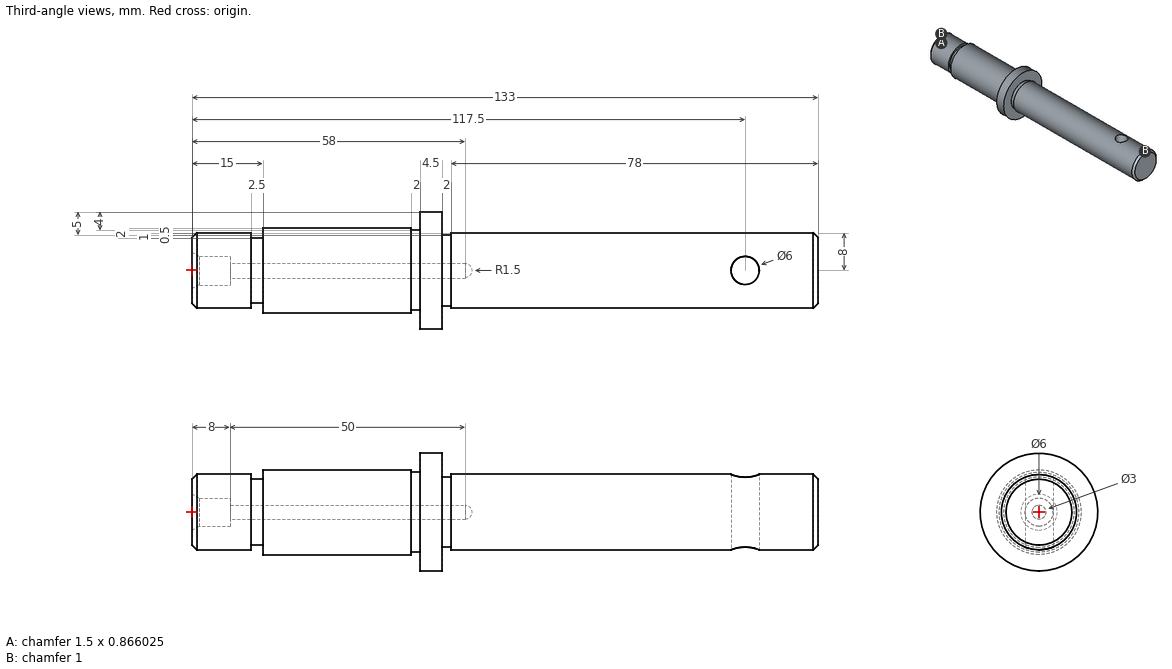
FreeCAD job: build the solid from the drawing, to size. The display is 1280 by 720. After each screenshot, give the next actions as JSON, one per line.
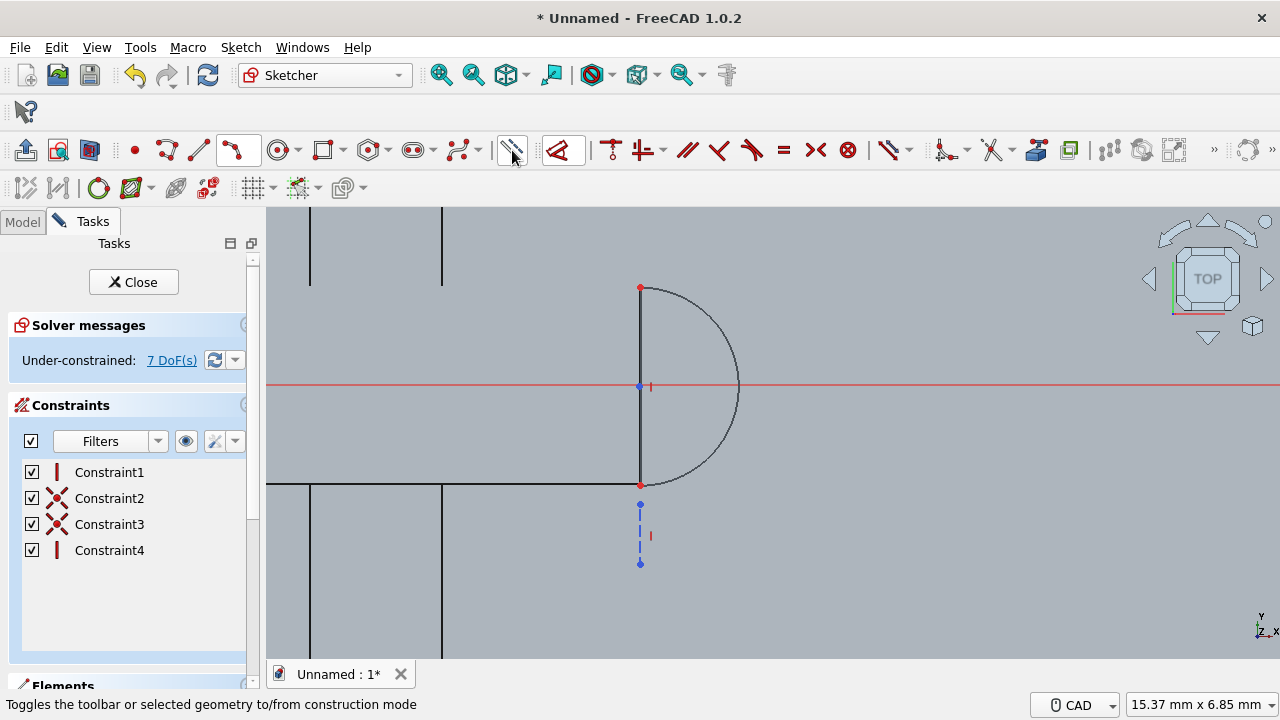
{"action": "left_click", "coordinate": [640, 387]}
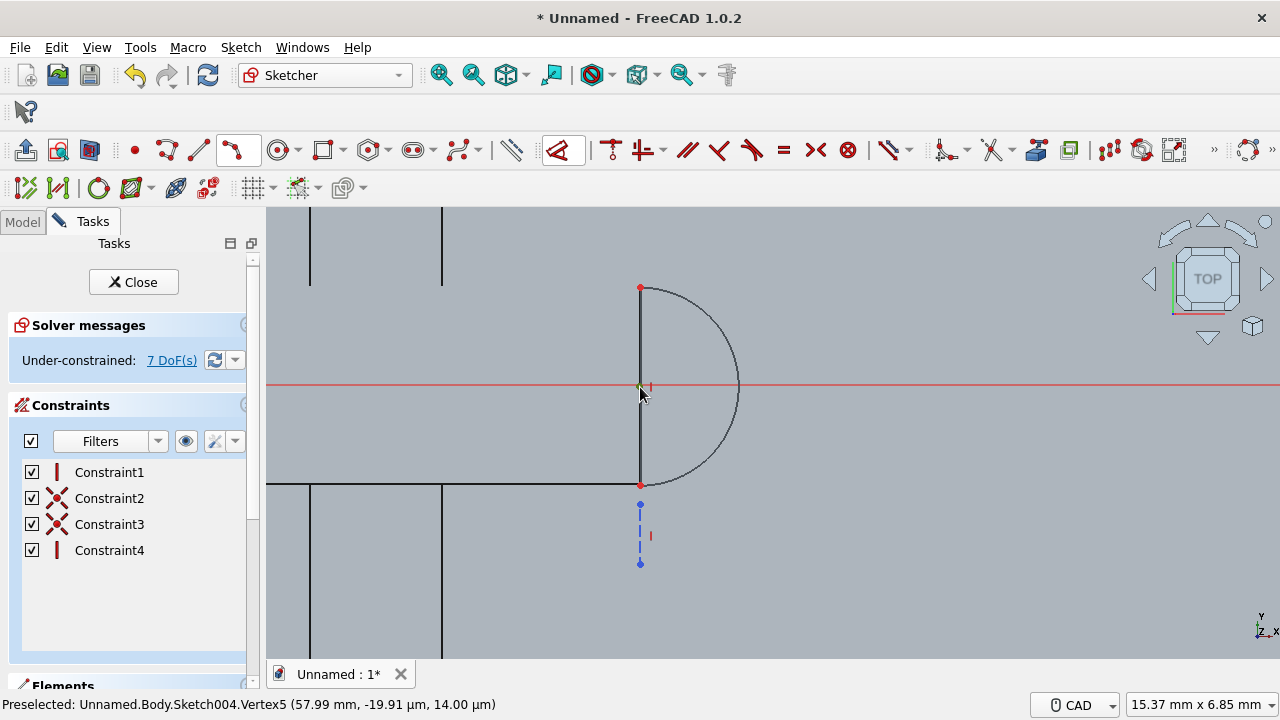
{"action": "left_click", "coordinate": [353, 385]}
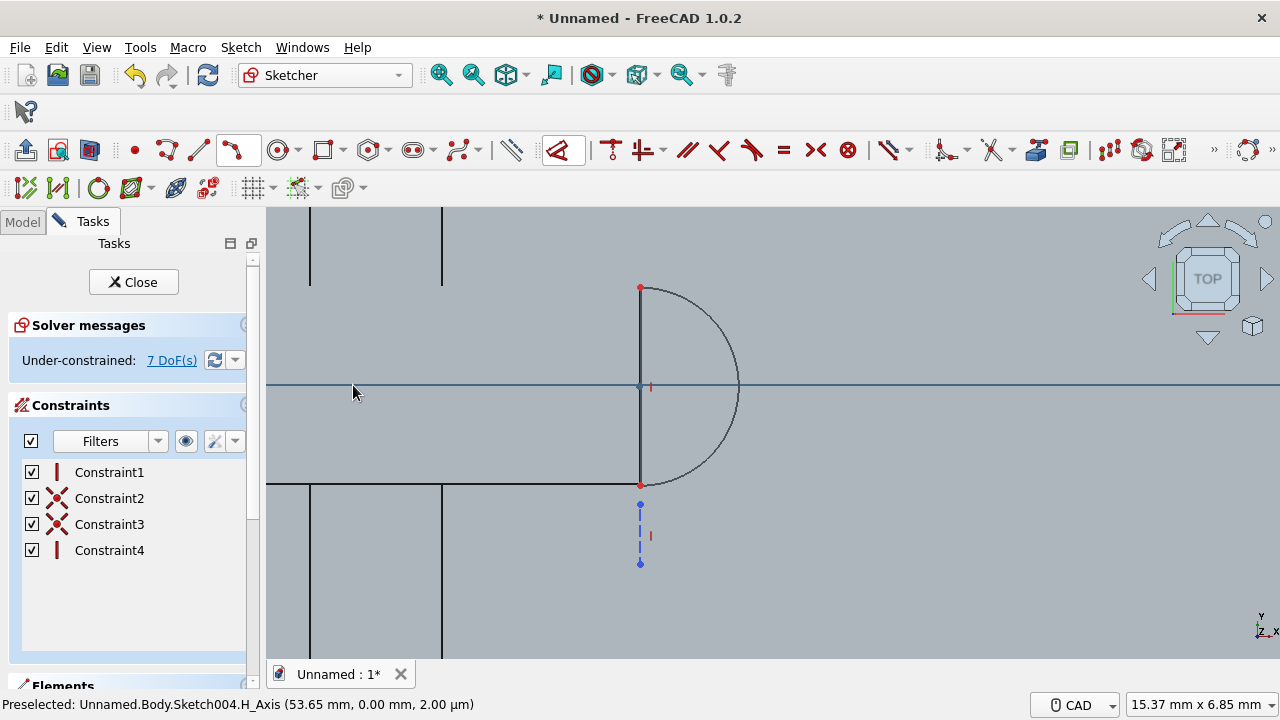
{"action": "key", "text": "c"}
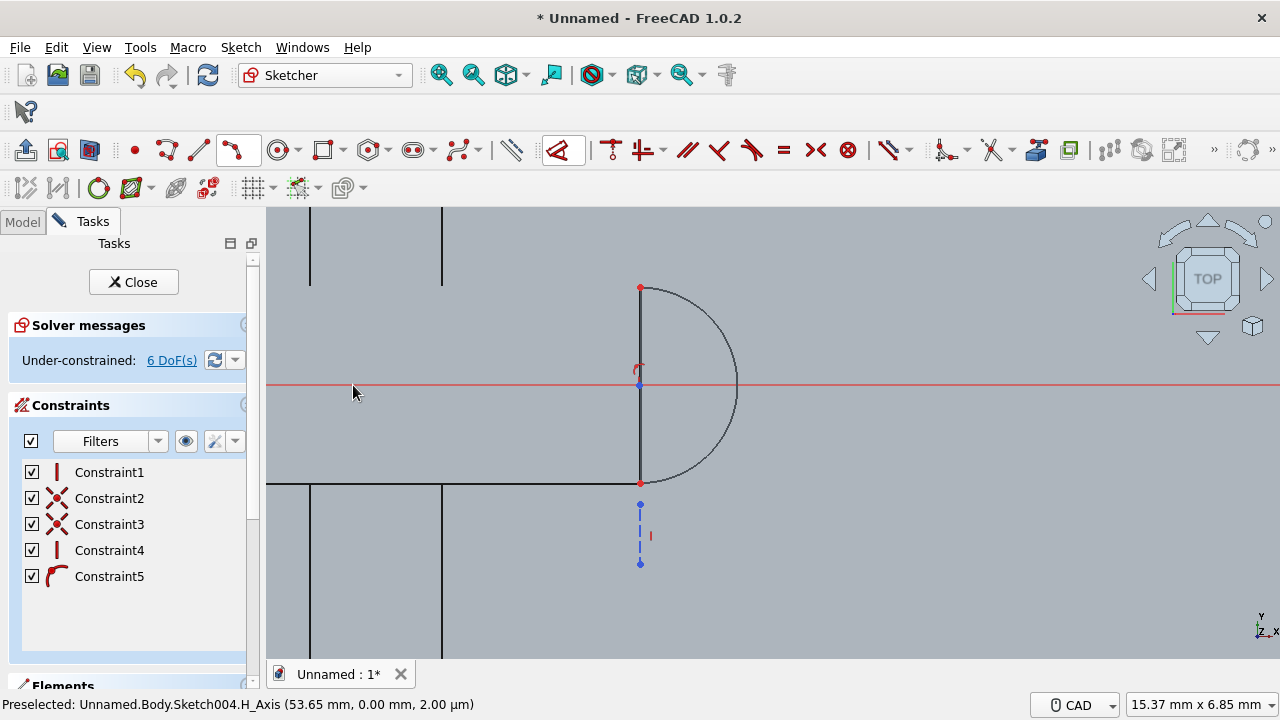
{"action": "left_click", "coordinate": [719, 443]}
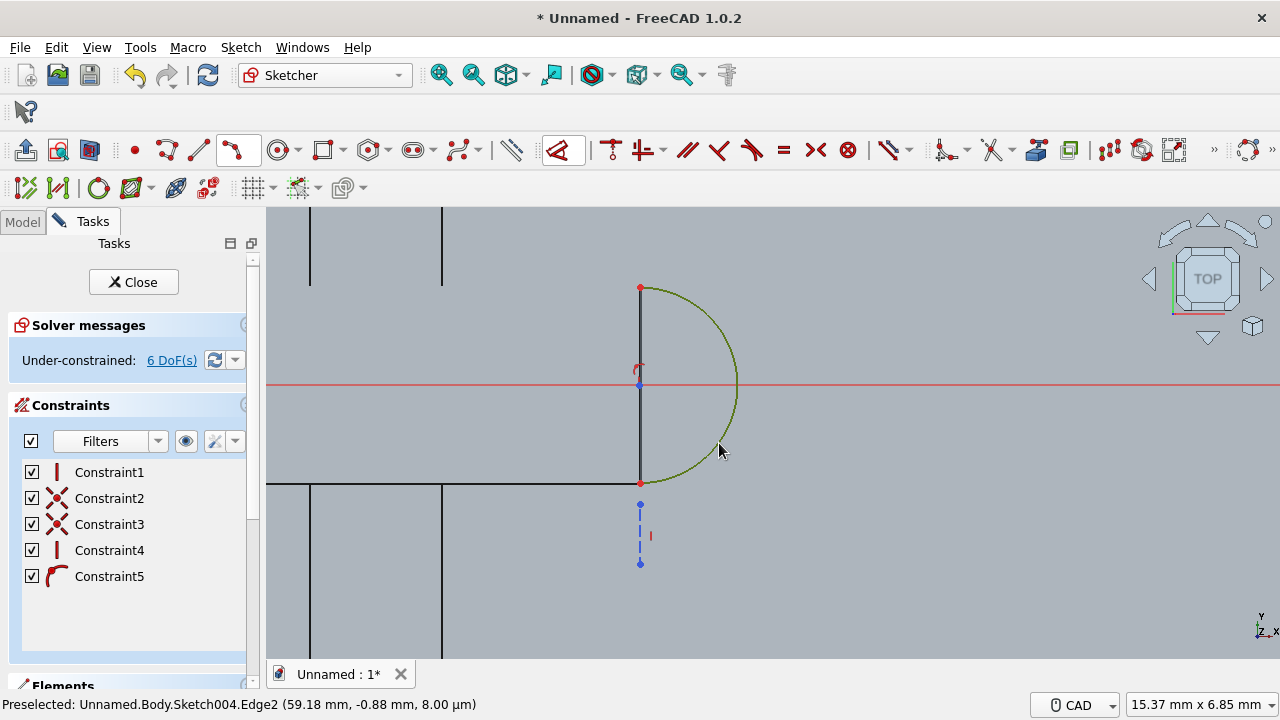
{"action": "left_click", "coordinate": [580, 150]}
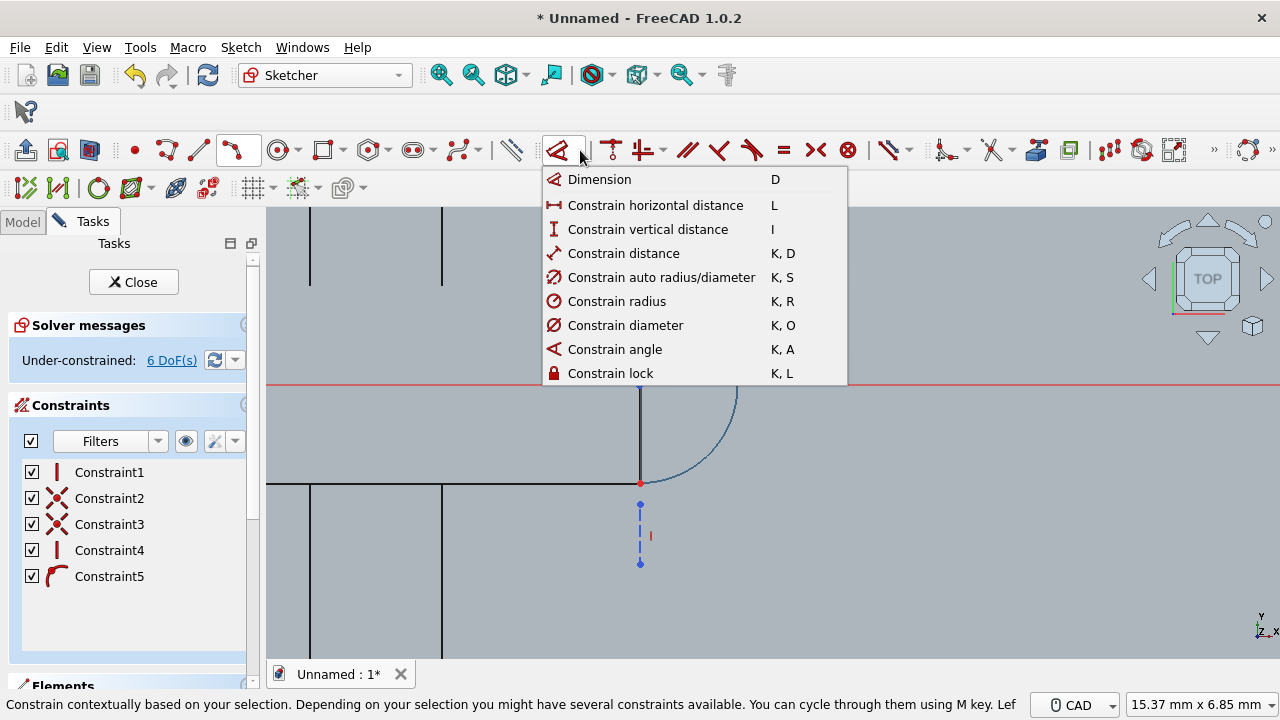
{"action": "left_click", "coordinate": [695, 301]}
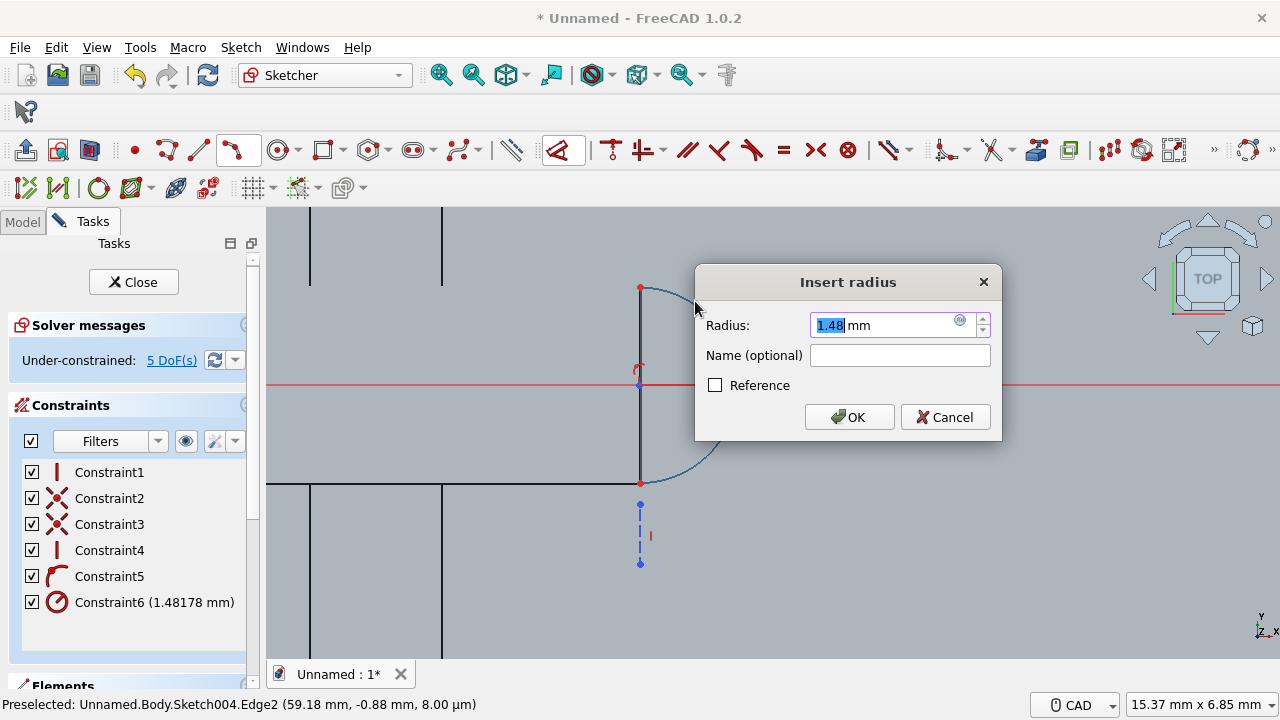
{"action": "type", "text": "1.5"}
{"action": "key", "text": "Return"}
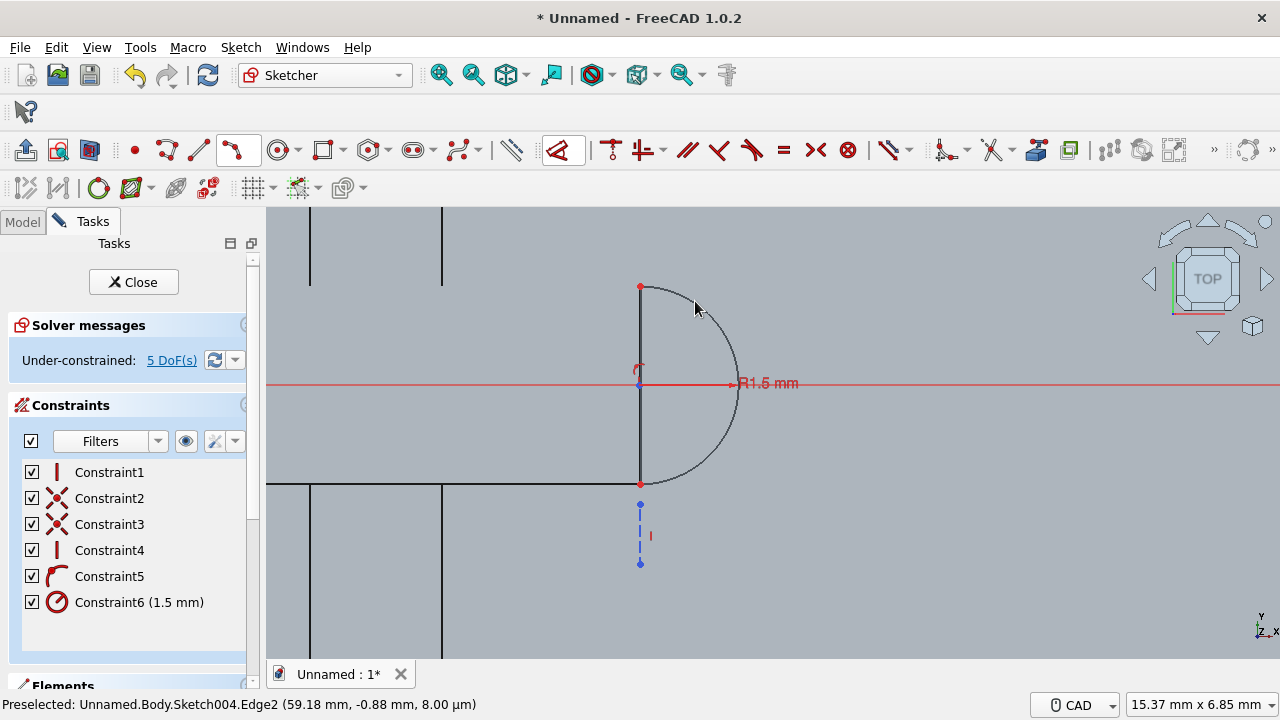
{"action": "left_click", "coordinate": [641, 286]}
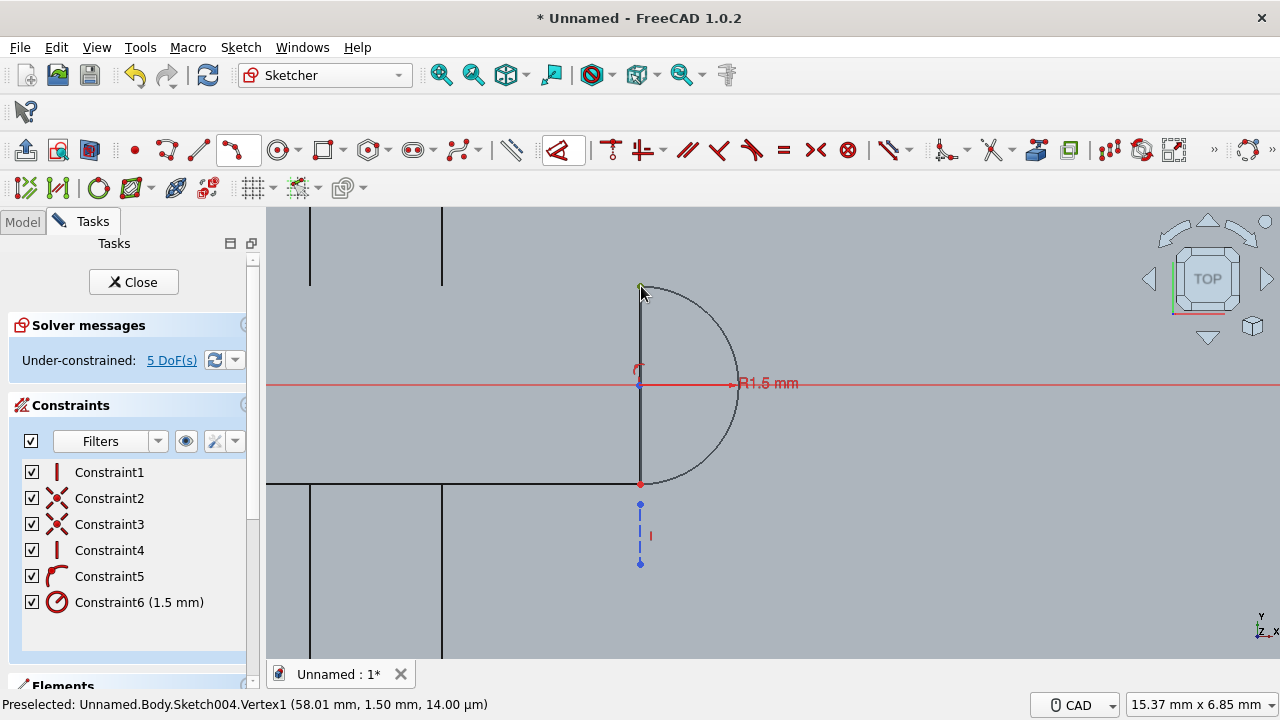
{"action": "left_click", "coordinate": [580, 150]}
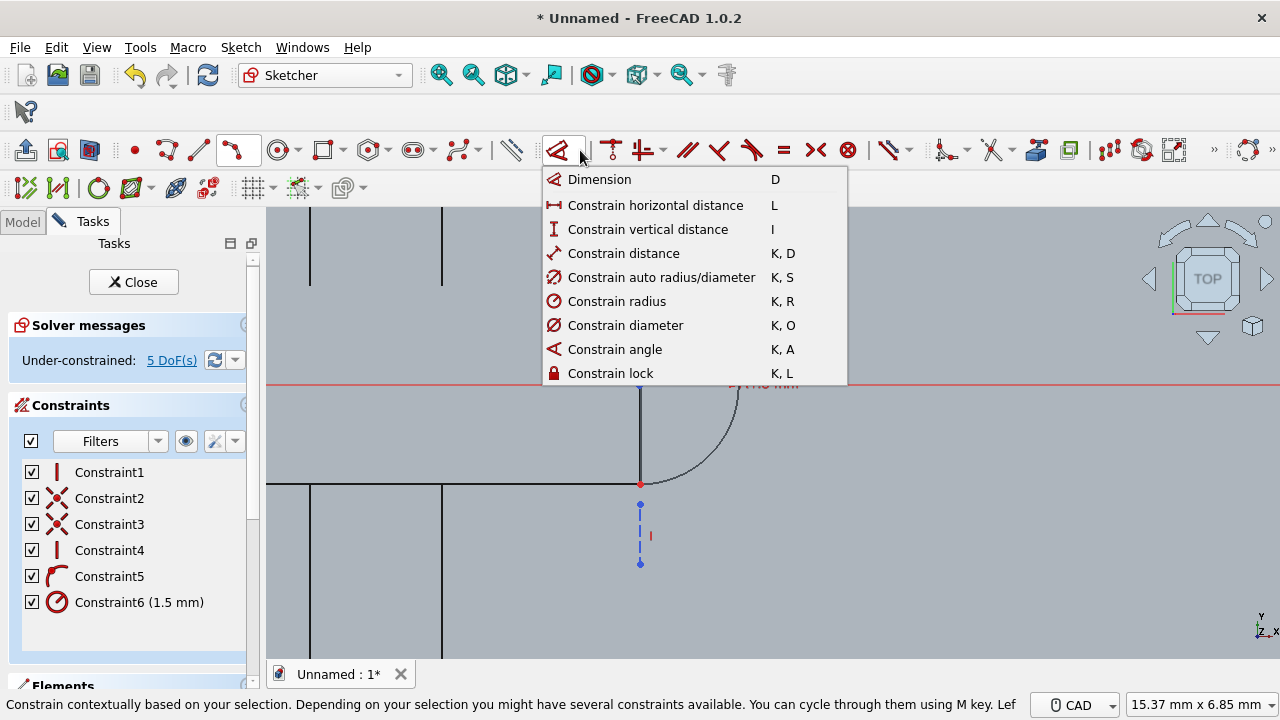
{"action": "left_click", "coordinate": [695, 205]}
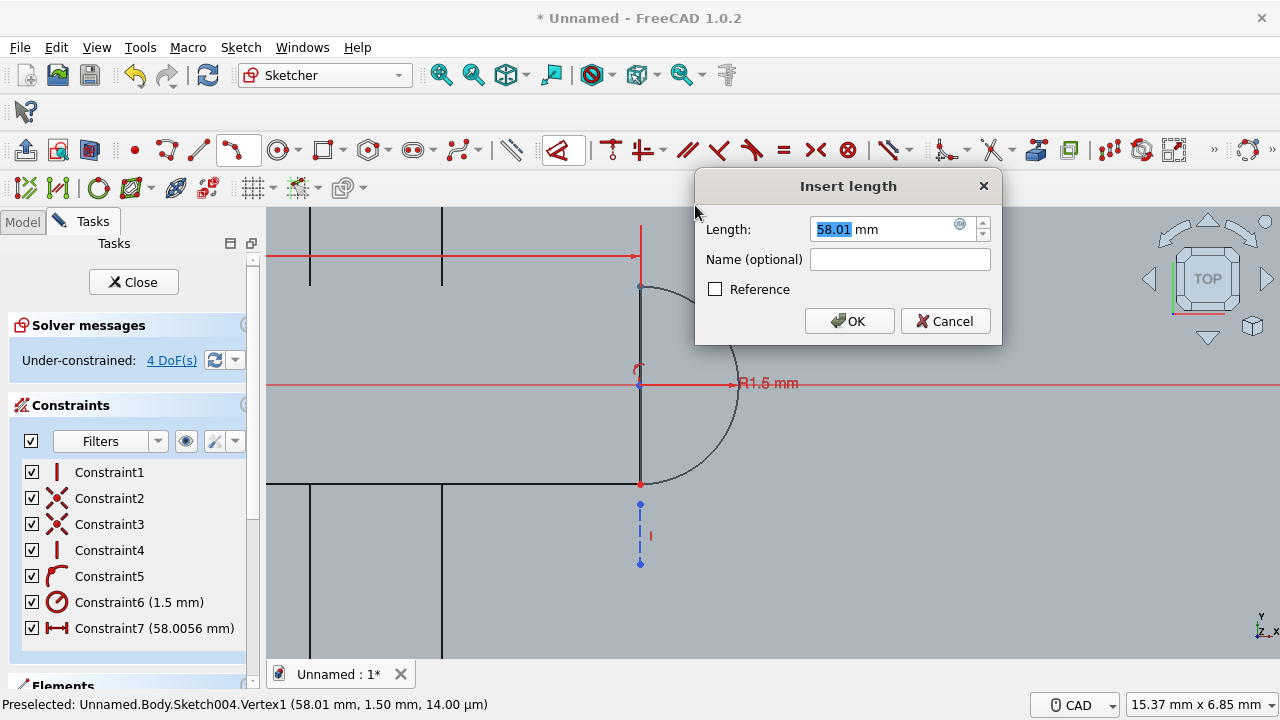
{"action": "type", "text": "58"}
{"action": "key", "text": "Return"}